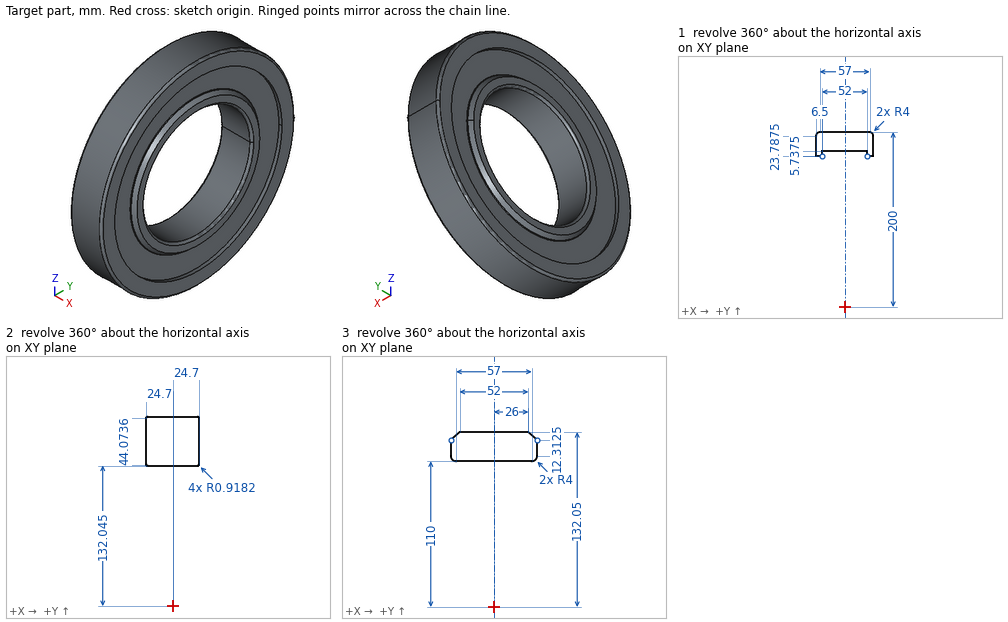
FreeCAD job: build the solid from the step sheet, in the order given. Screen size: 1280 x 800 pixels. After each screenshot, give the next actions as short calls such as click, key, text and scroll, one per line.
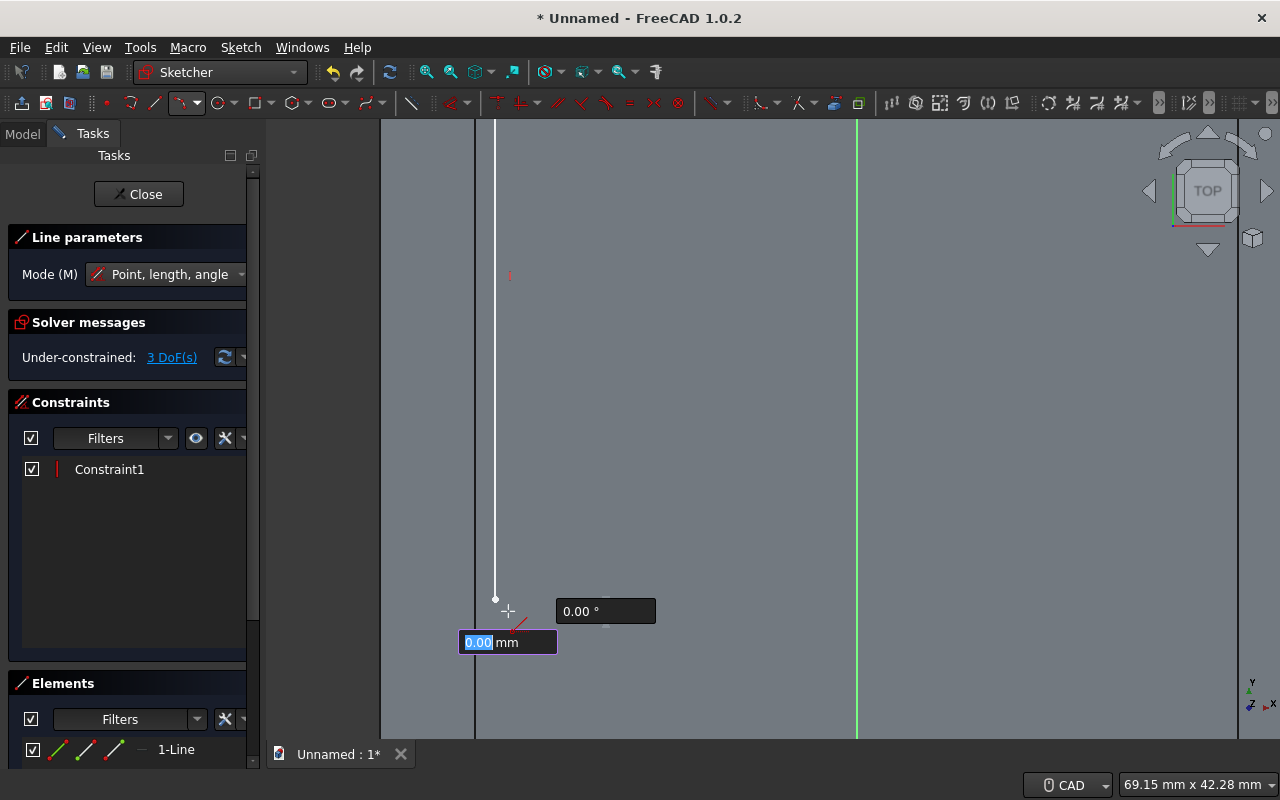
scroll(519, 617, down, 3)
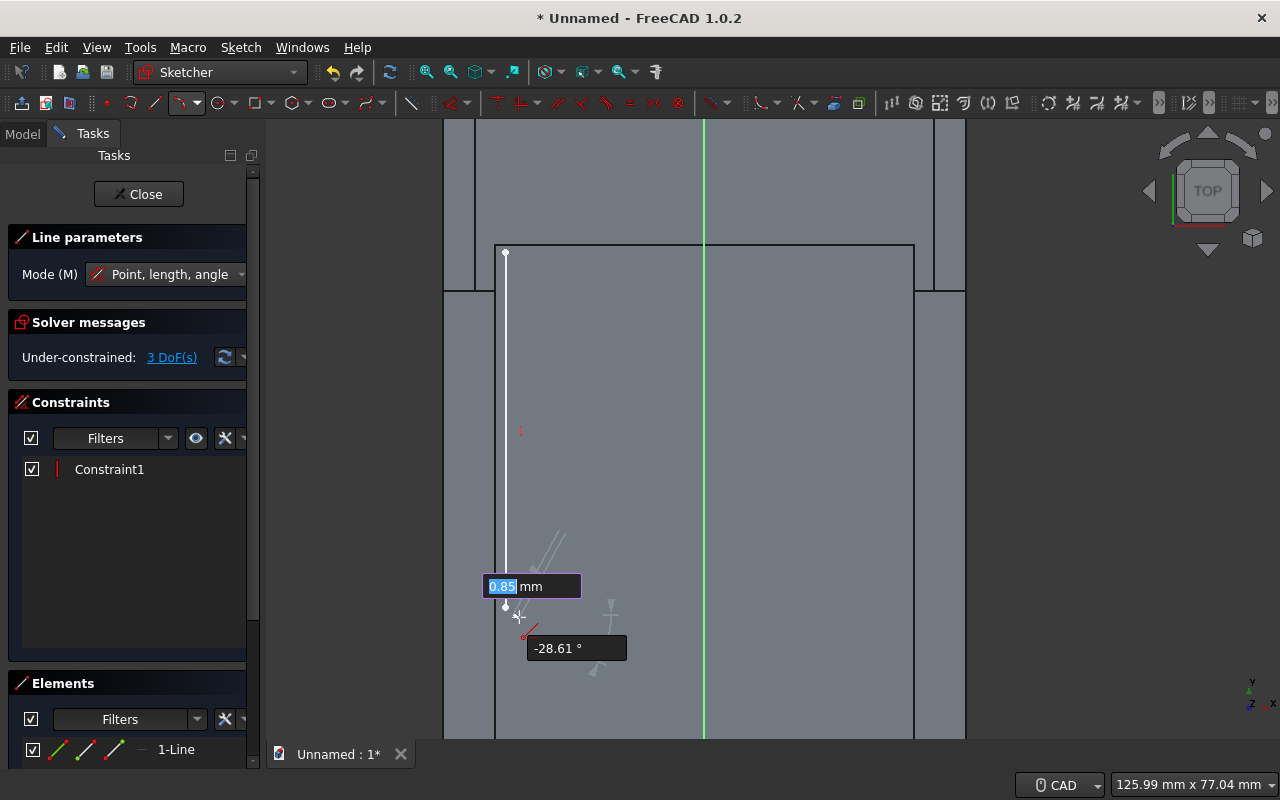
click(896, 614)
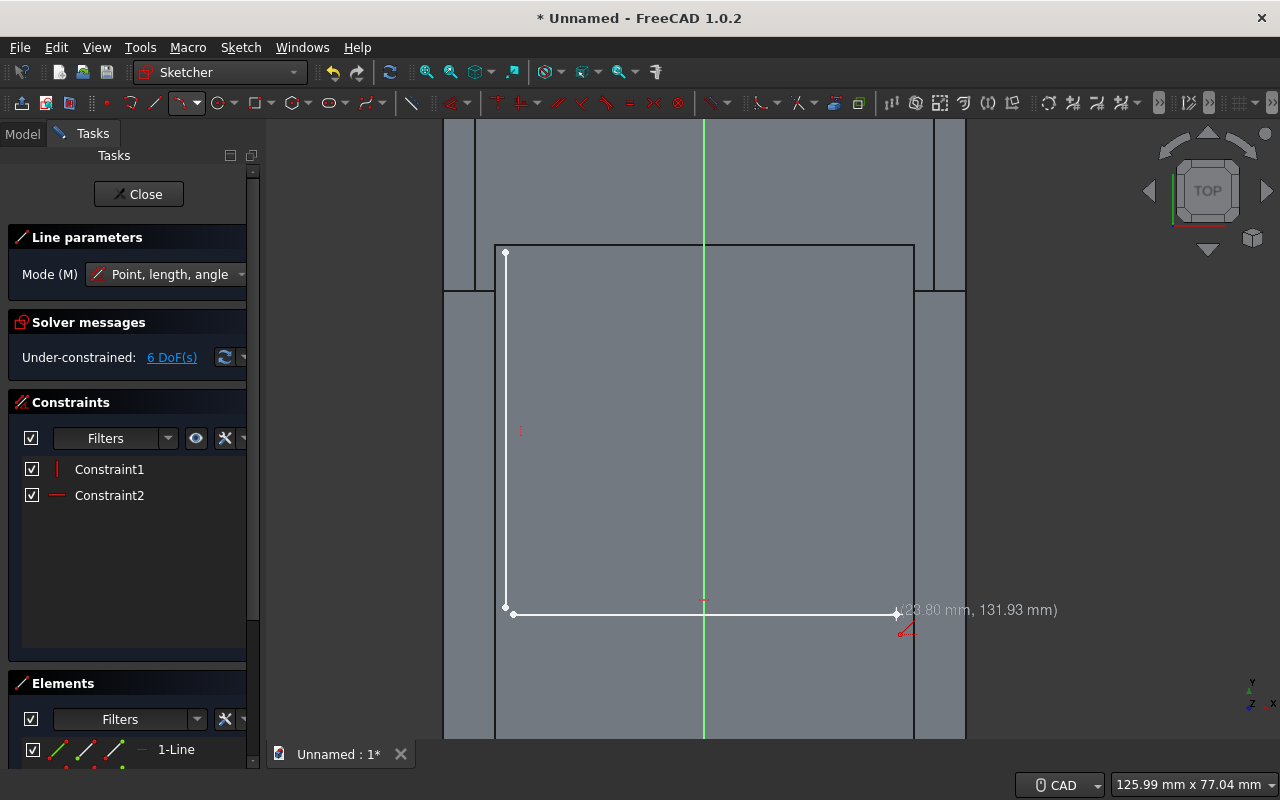
scroll(903, 607, up, 3)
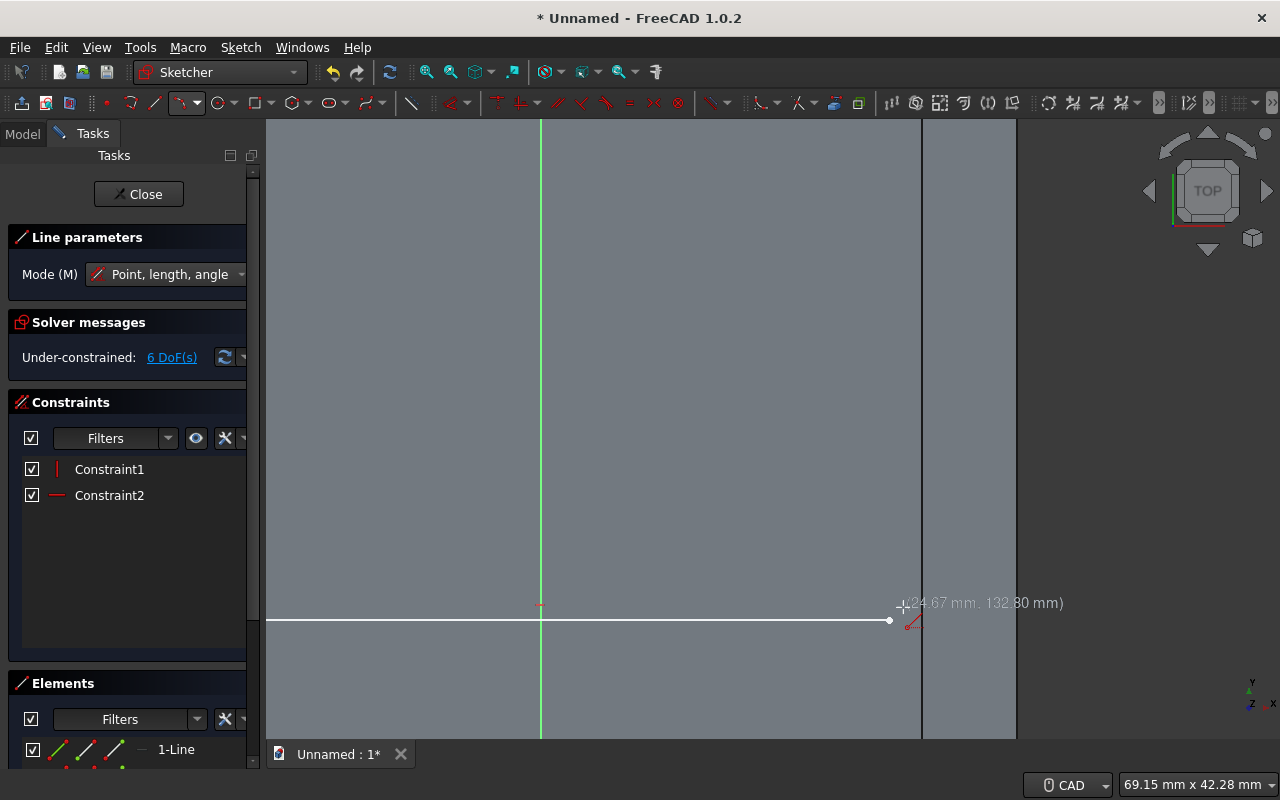
click(903, 606)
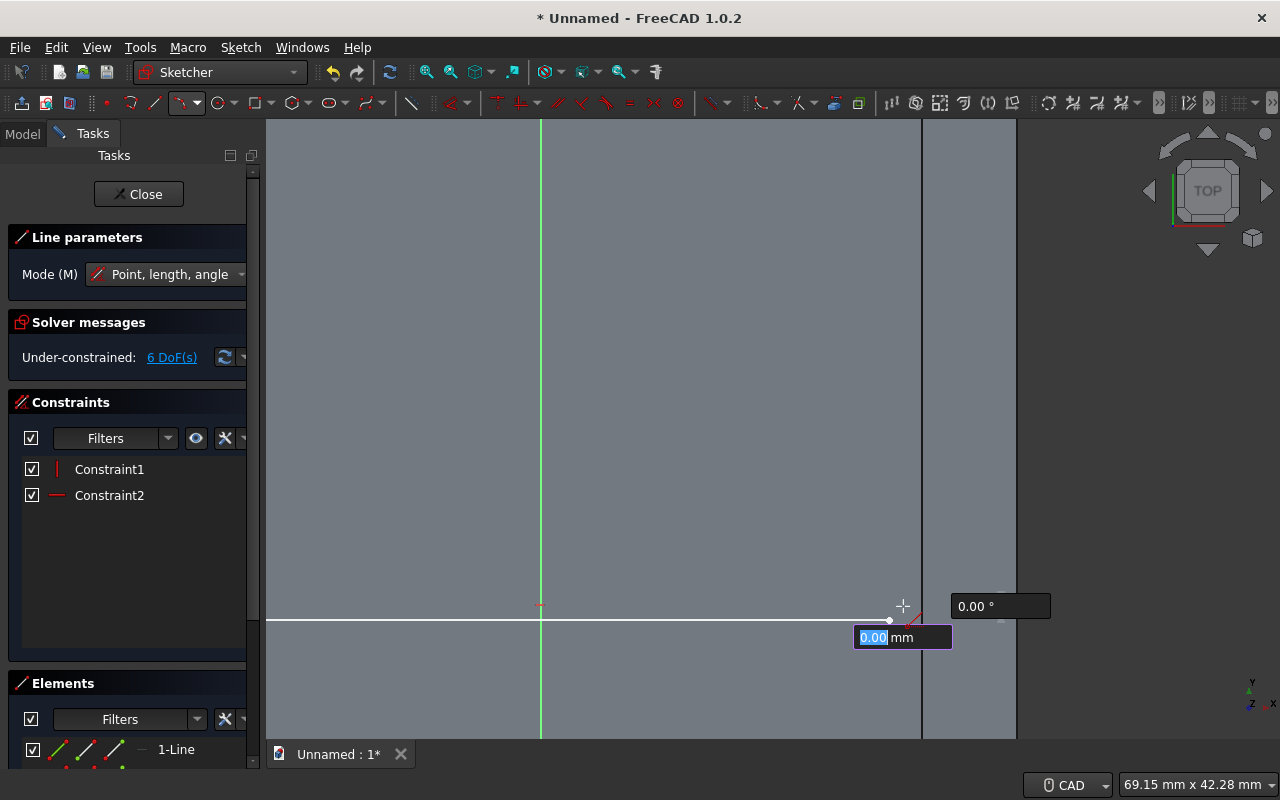
scroll(904, 607, down, 3)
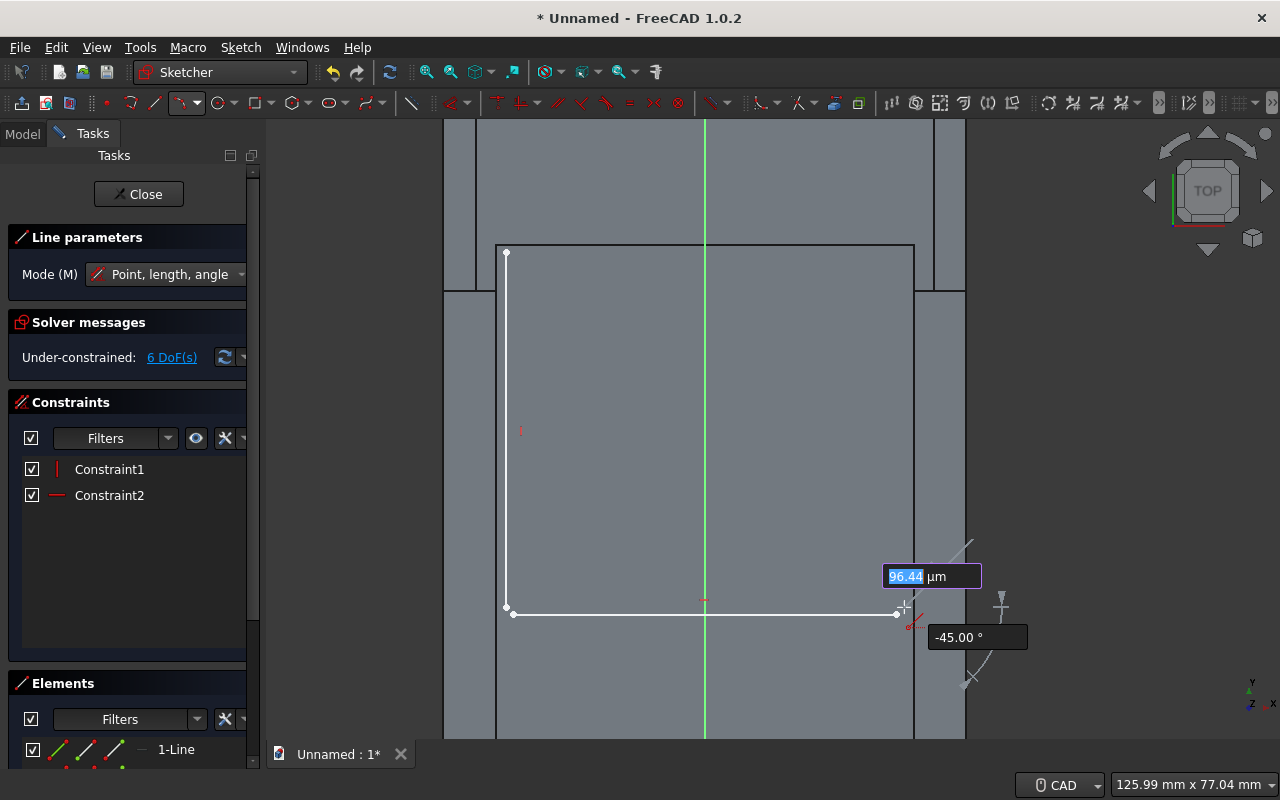
click(904, 252)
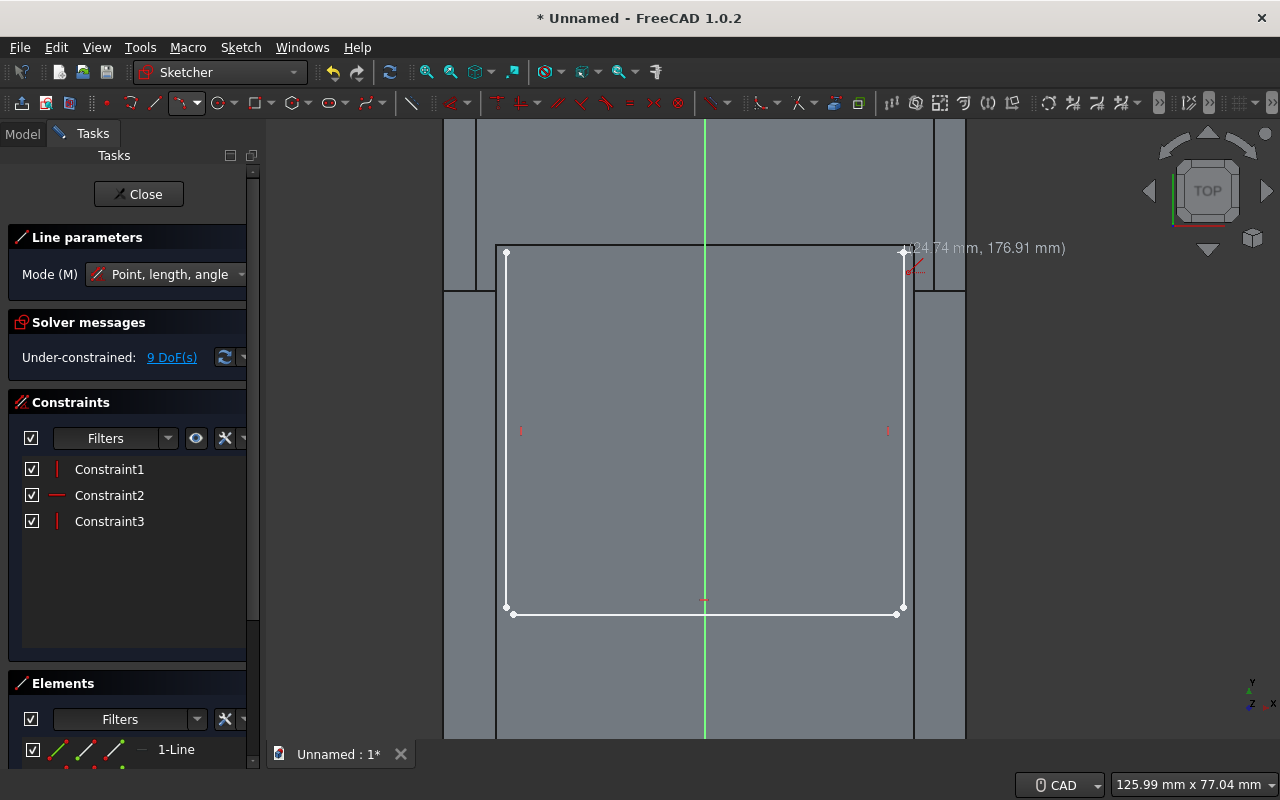
scroll(896, 245, up, 3)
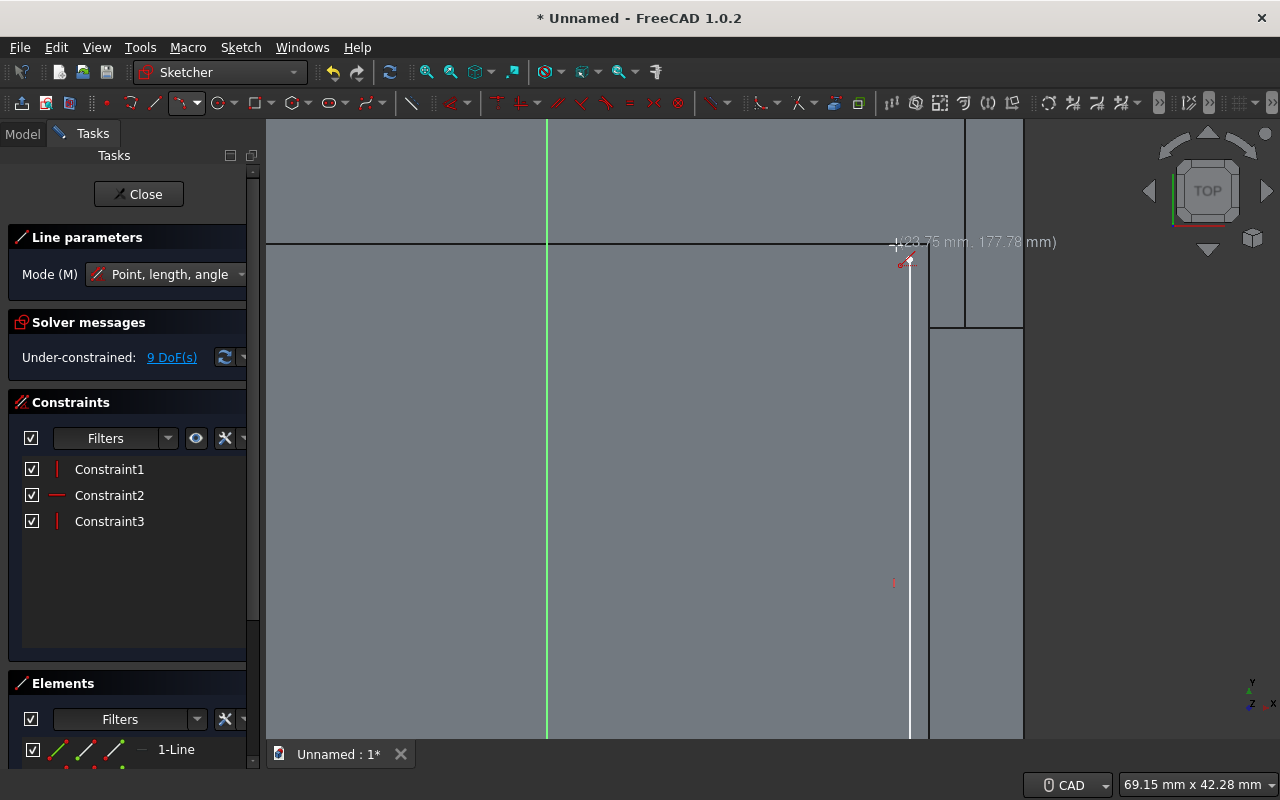
click(896, 244)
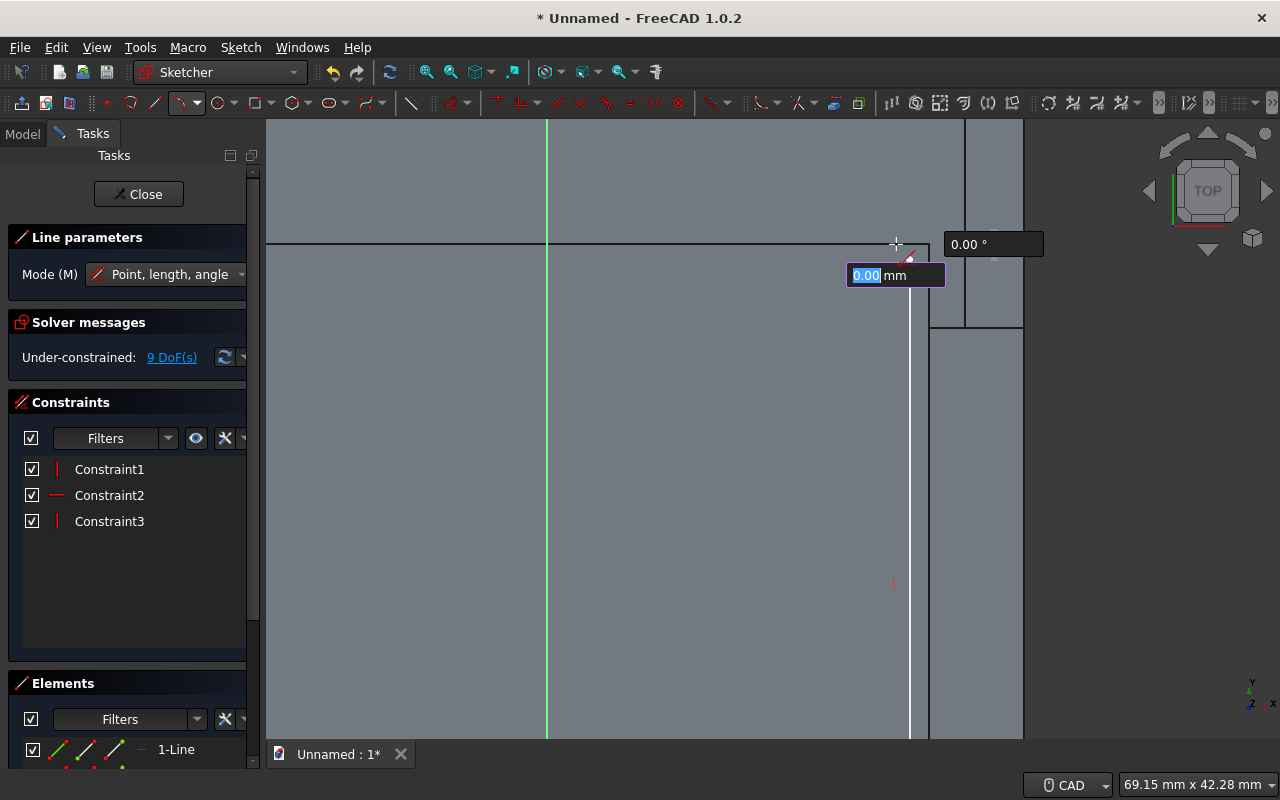
scroll(896, 244, down, 3)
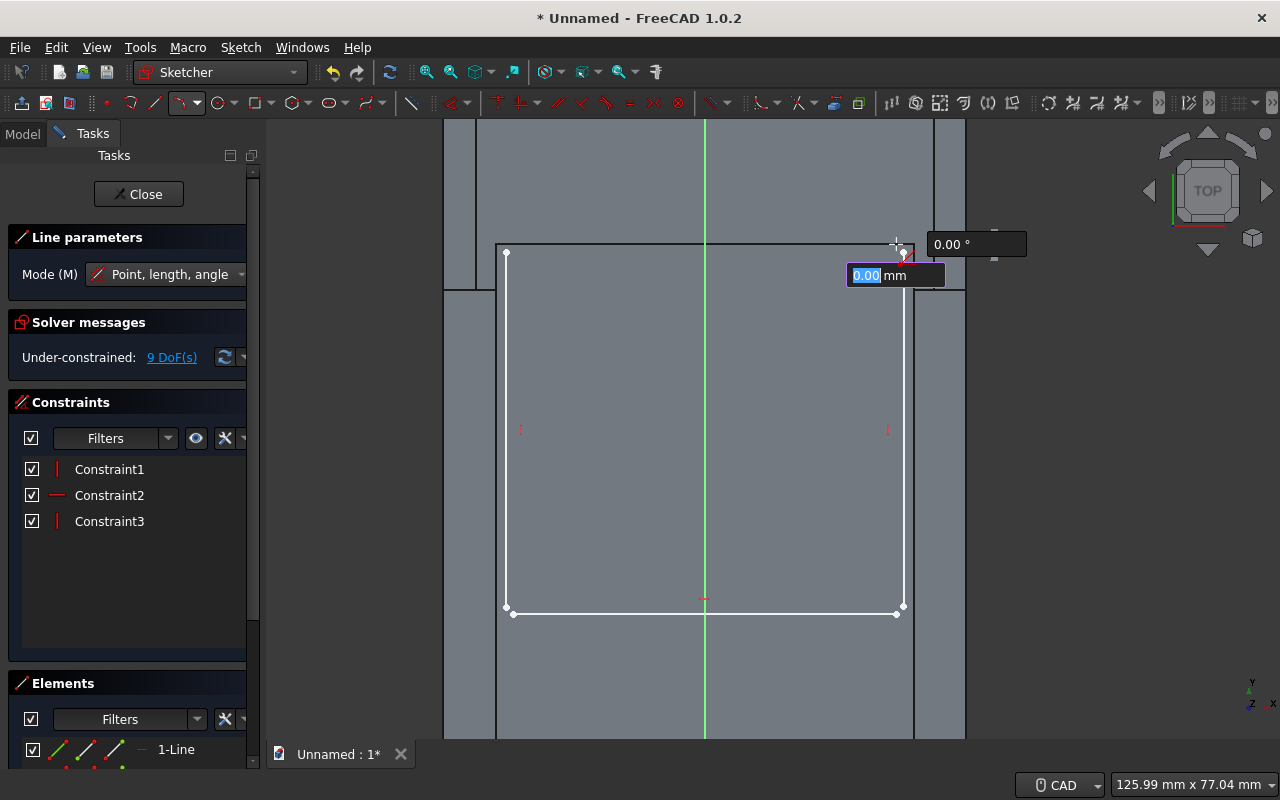
scroll(513, 244, up, 3)